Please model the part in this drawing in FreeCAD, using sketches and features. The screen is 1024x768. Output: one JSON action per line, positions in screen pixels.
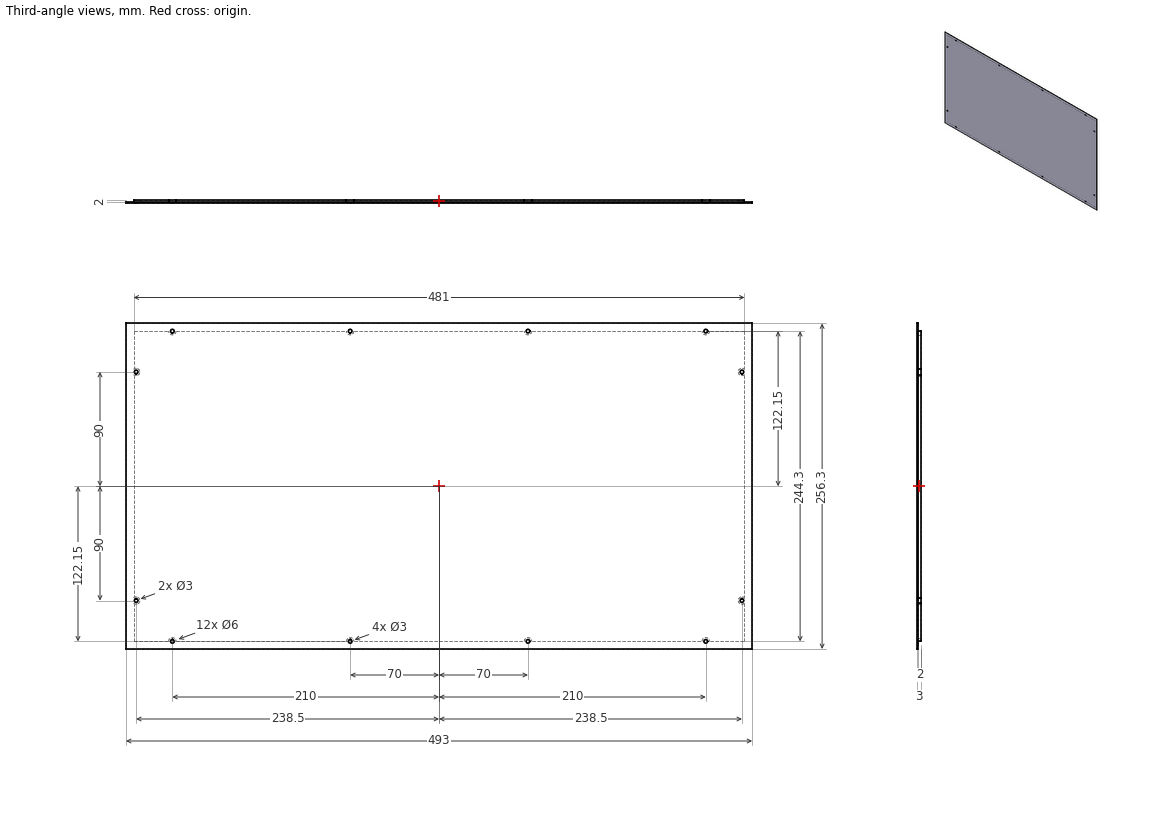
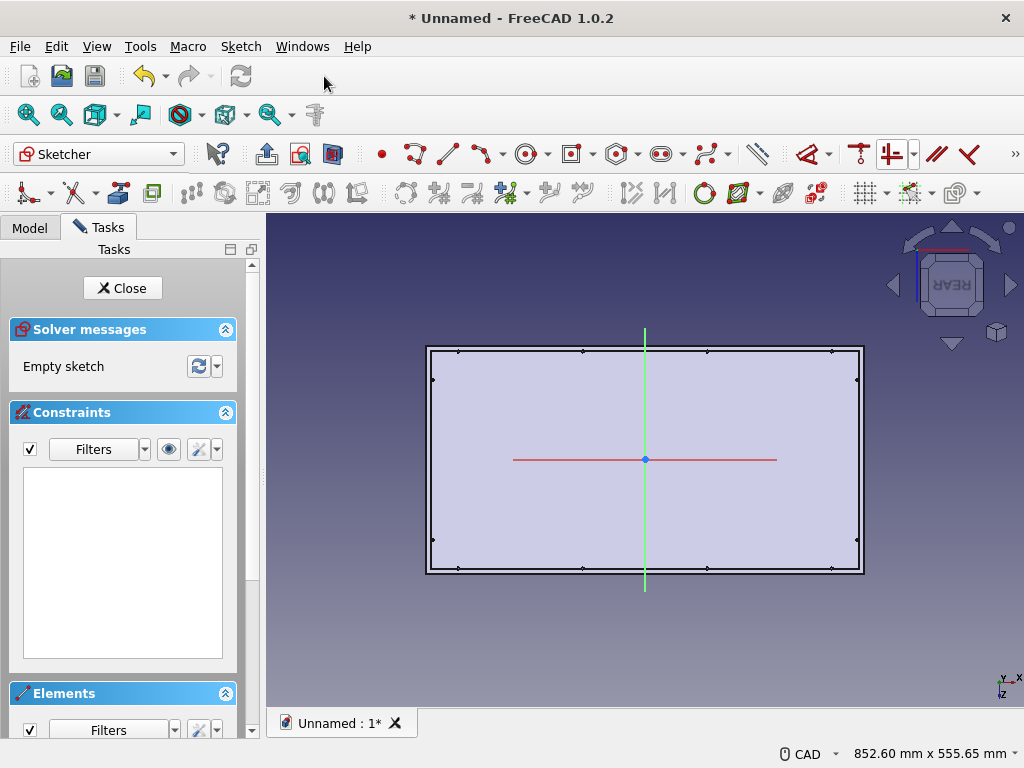
{"action": "scroll", "coordinate": [294, 460], "scroll_direction": "down", "scroll_amount": 1}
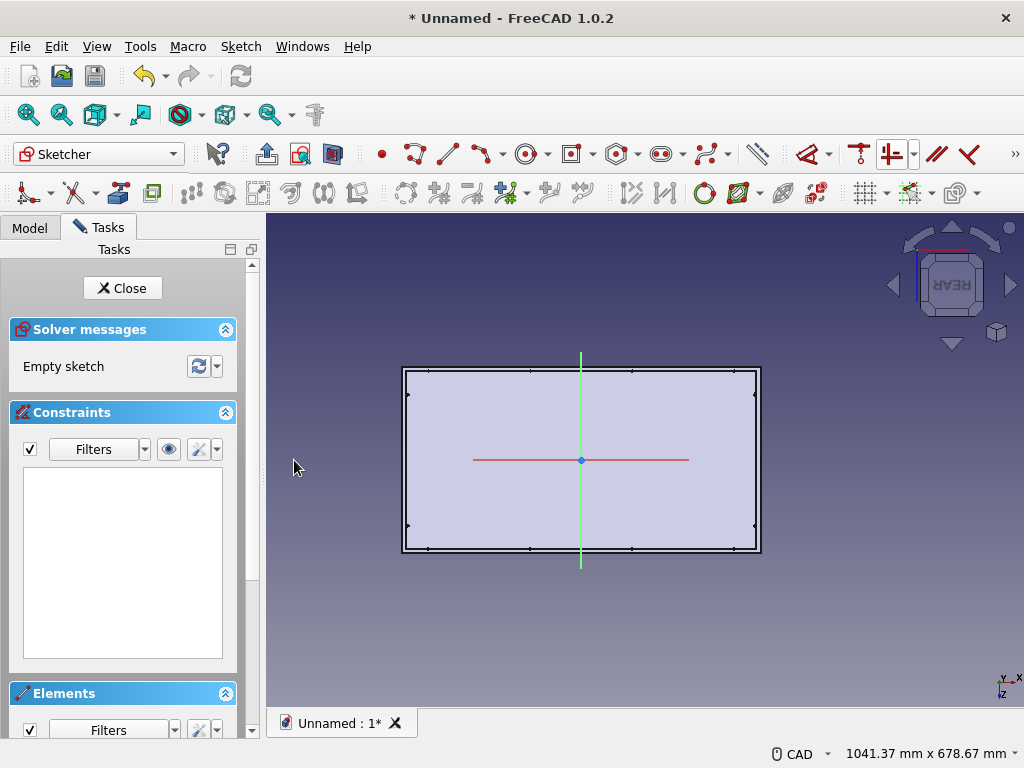
{"action": "left_click", "coordinate": [526, 154]}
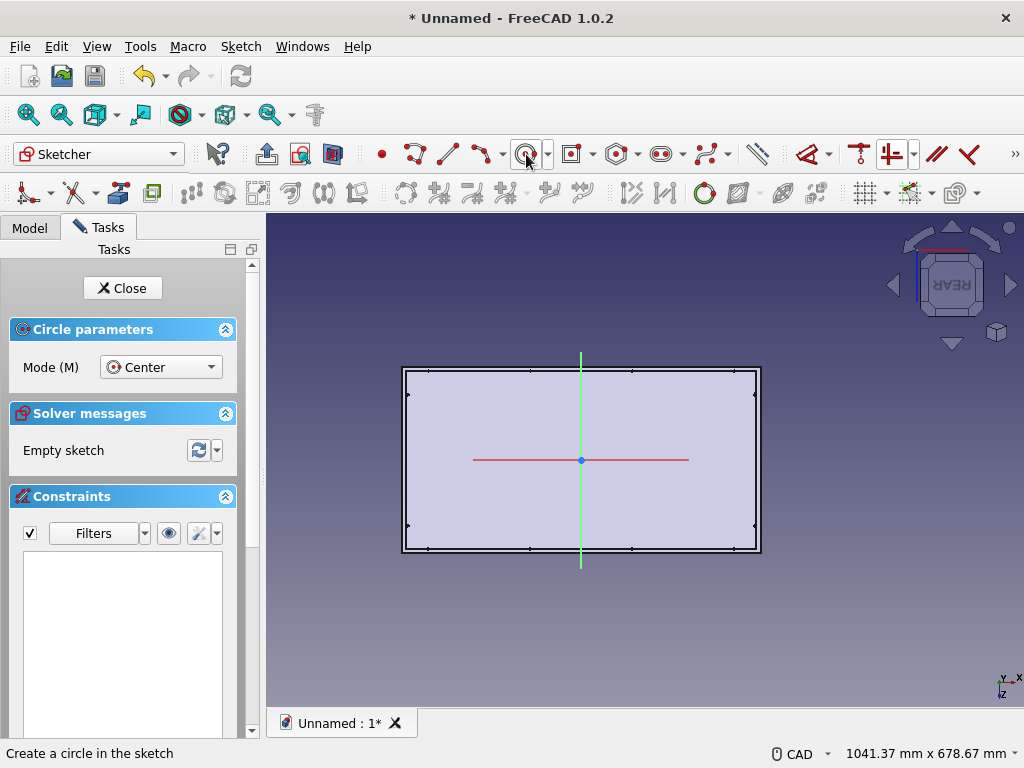
{"action": "scroll", "coordinate": [429, 371], "scroll_direction": "up", "scroll_amount": 12}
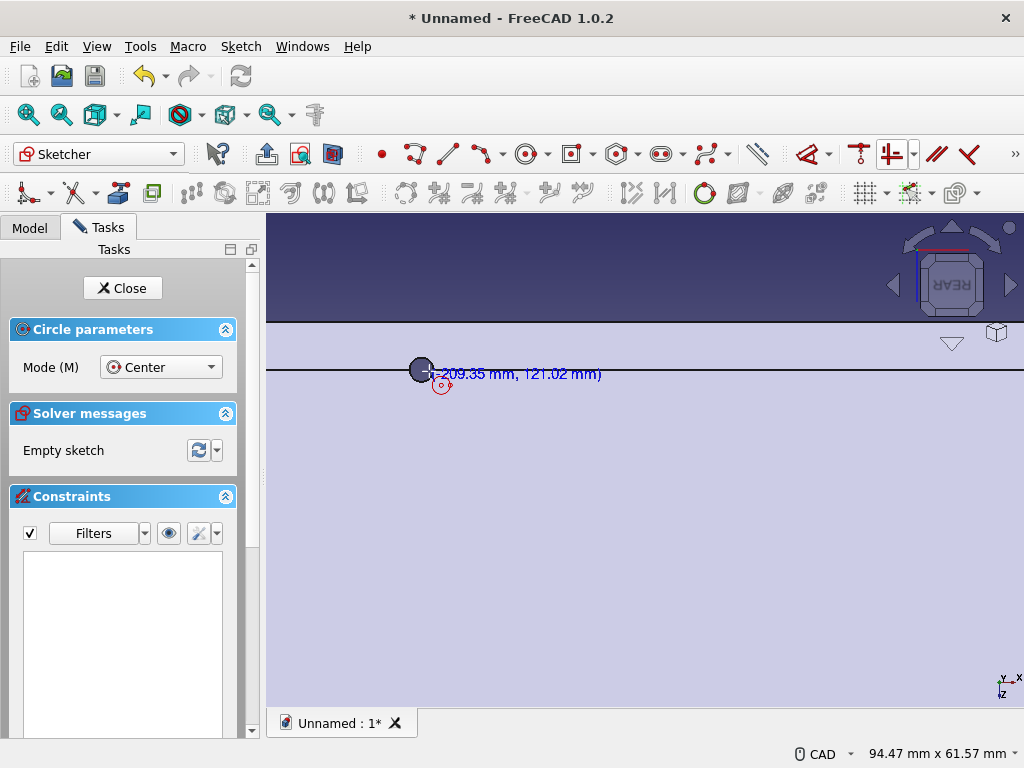
{"action": "scroll", "coordinate": [386, 349], "scroll_direction": "down", "scroll_amount": 11}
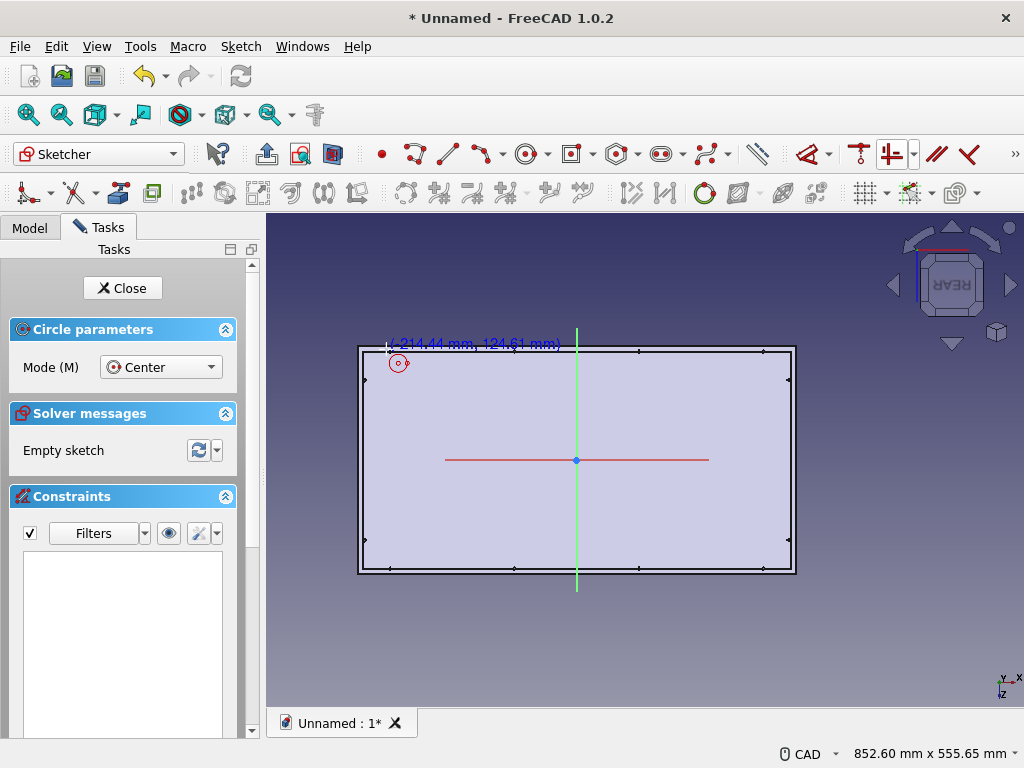
{"action": "left_click", "coordinate": [390, 352]}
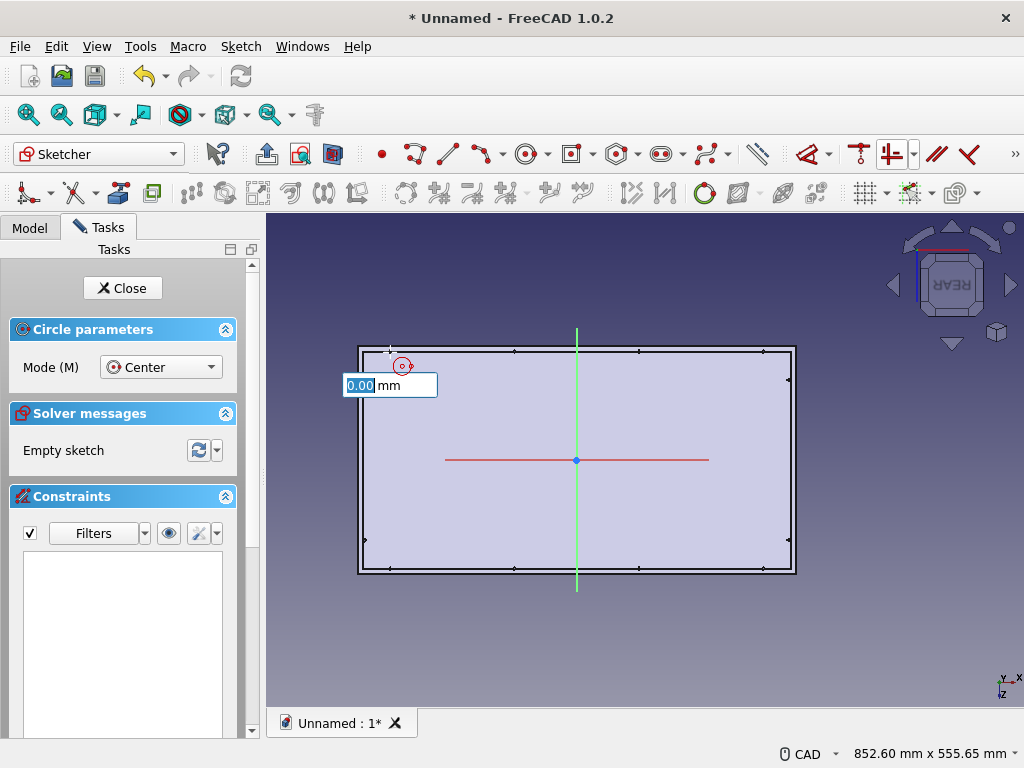
{"action": "scroll", "coordinate": [392, 350], "scroll_direction": "up", "scroll_amount": 9}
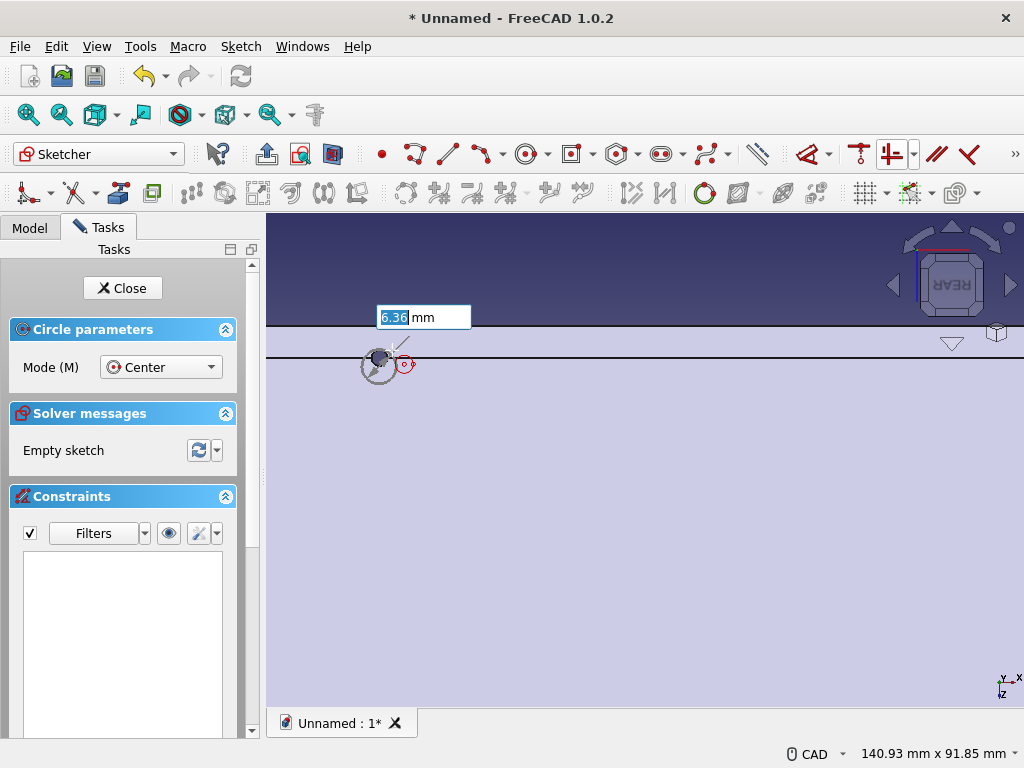
{"action": "left_click", "coordinate": [391, 347]}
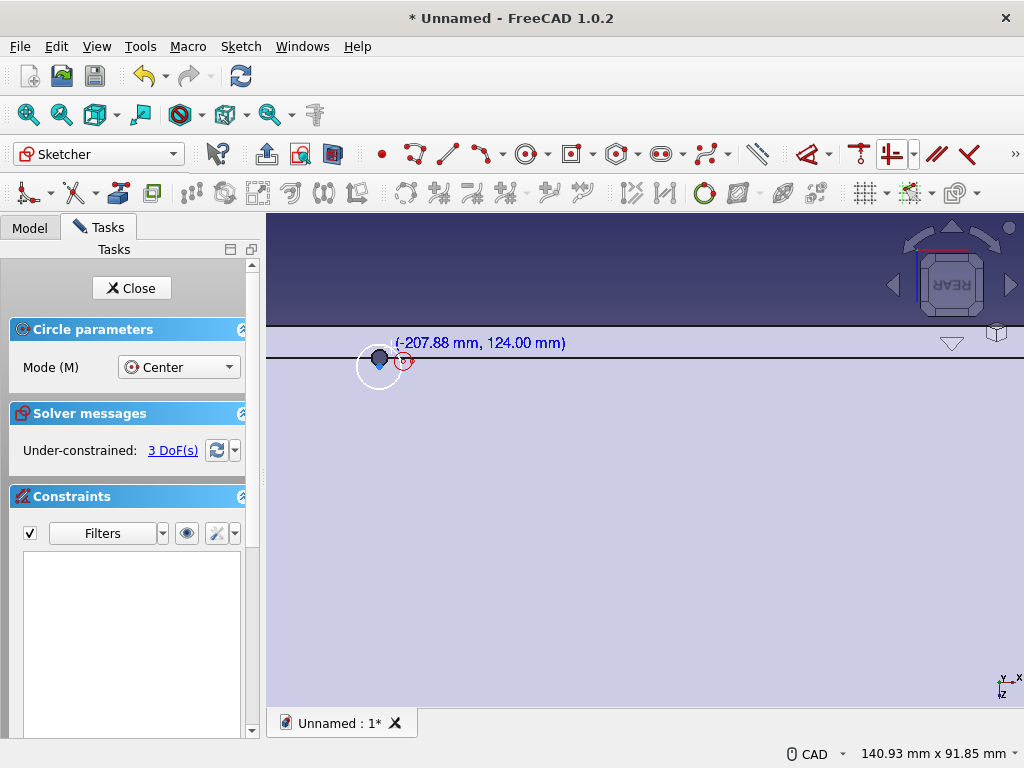
{"action": "scroll", "coordinate": [392, 350], "scroll_direction": "down", "scroll_amount": 9}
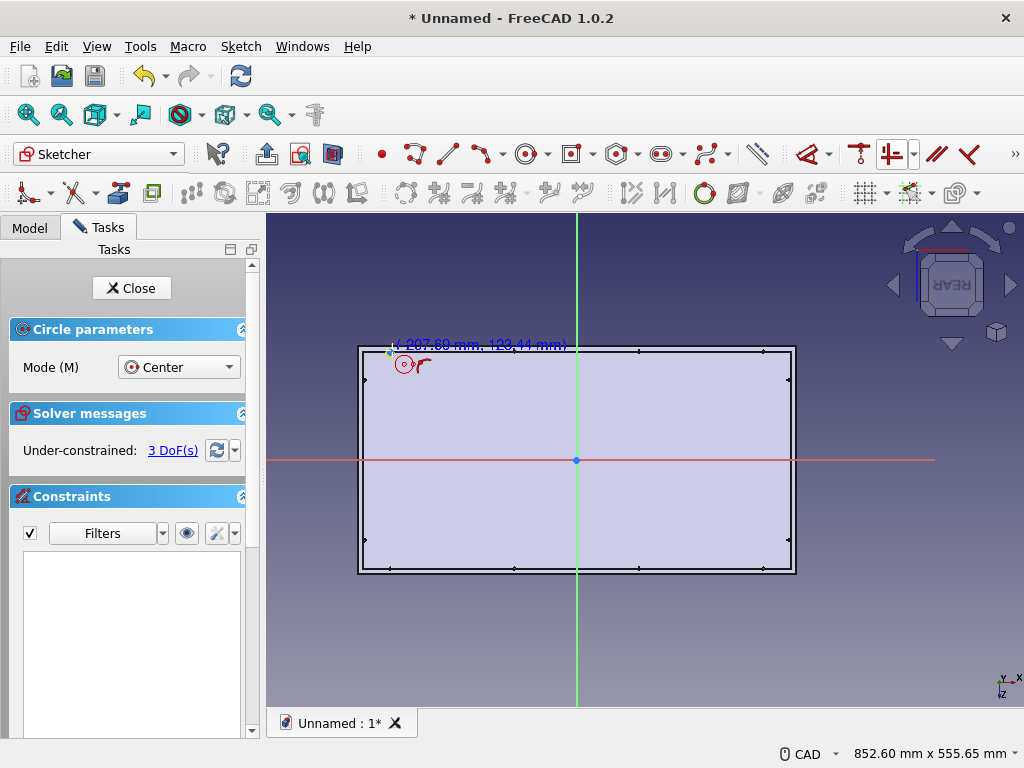
{"action": "scroll", "coordinate": [515, 352], "scroll_direction": "up", "scroll_amount": 11}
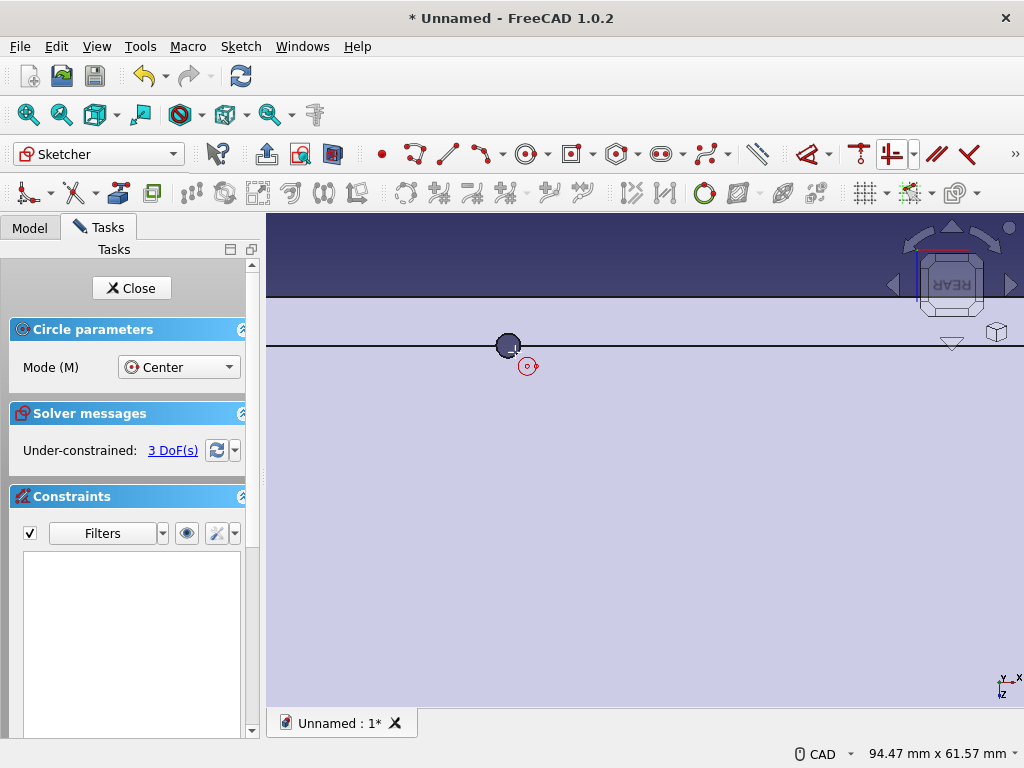
{"action": "scroll", "coordinate": [515, 352], "scroll_direction": "down", "scroll_amount": 11}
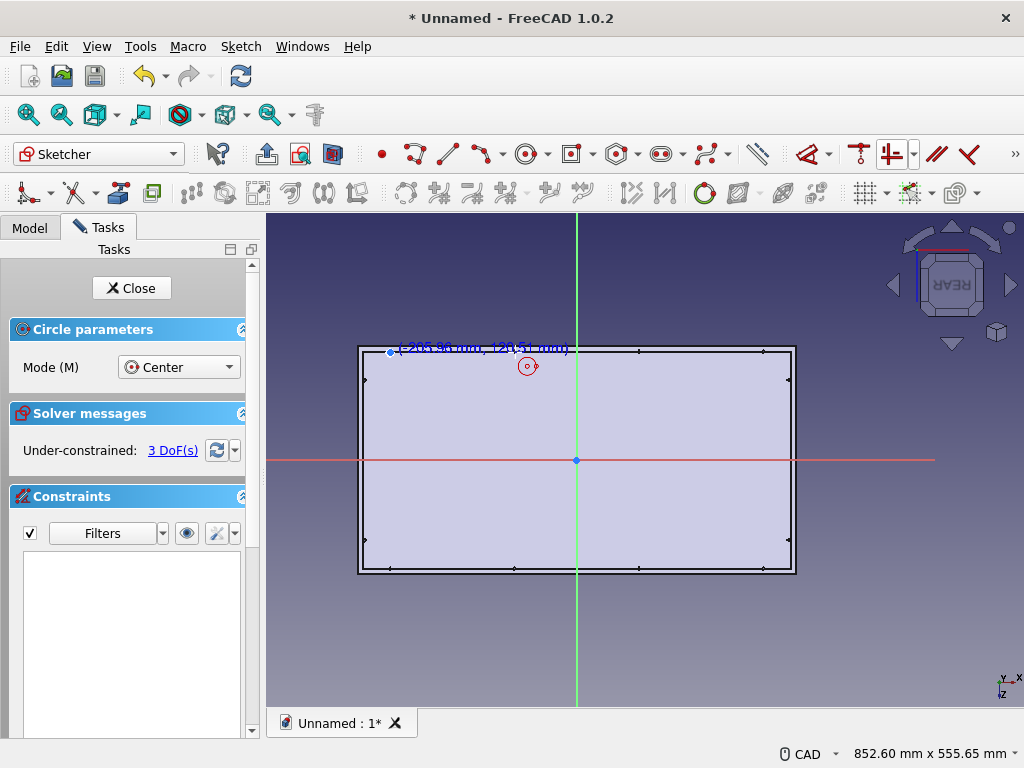
{"action": "left_click", "coordinate": [515, 352]}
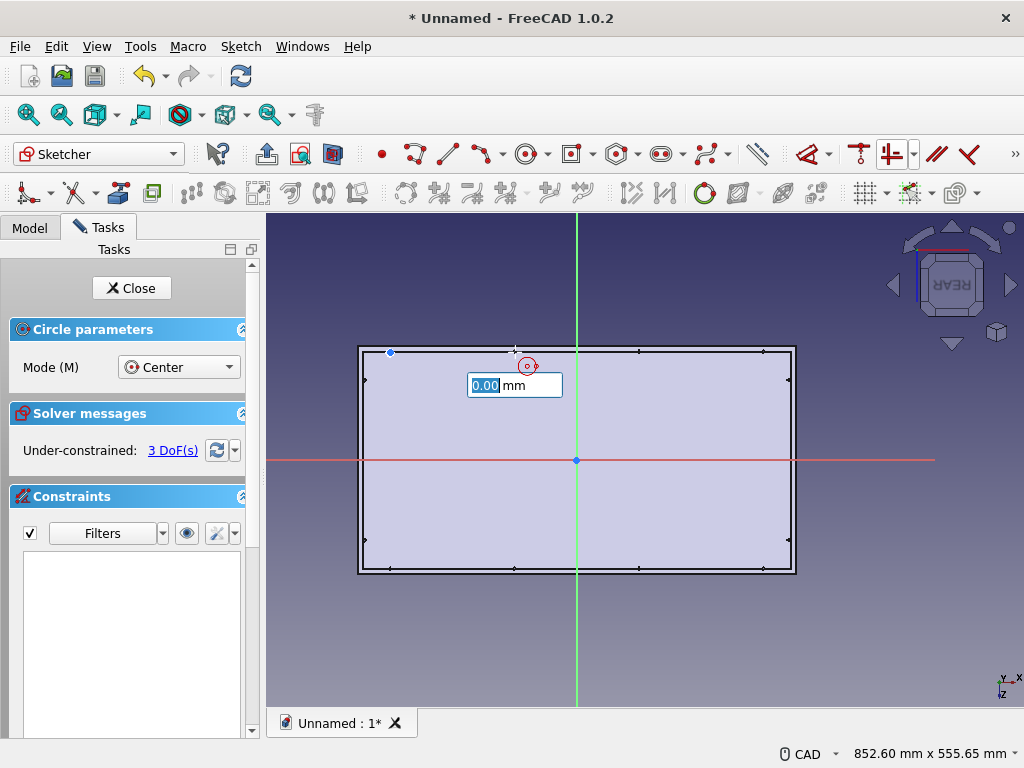
{"action": "scroll", "coordinate": [516, 350], "scroll_direction": "up", "scroll_amount": 9}